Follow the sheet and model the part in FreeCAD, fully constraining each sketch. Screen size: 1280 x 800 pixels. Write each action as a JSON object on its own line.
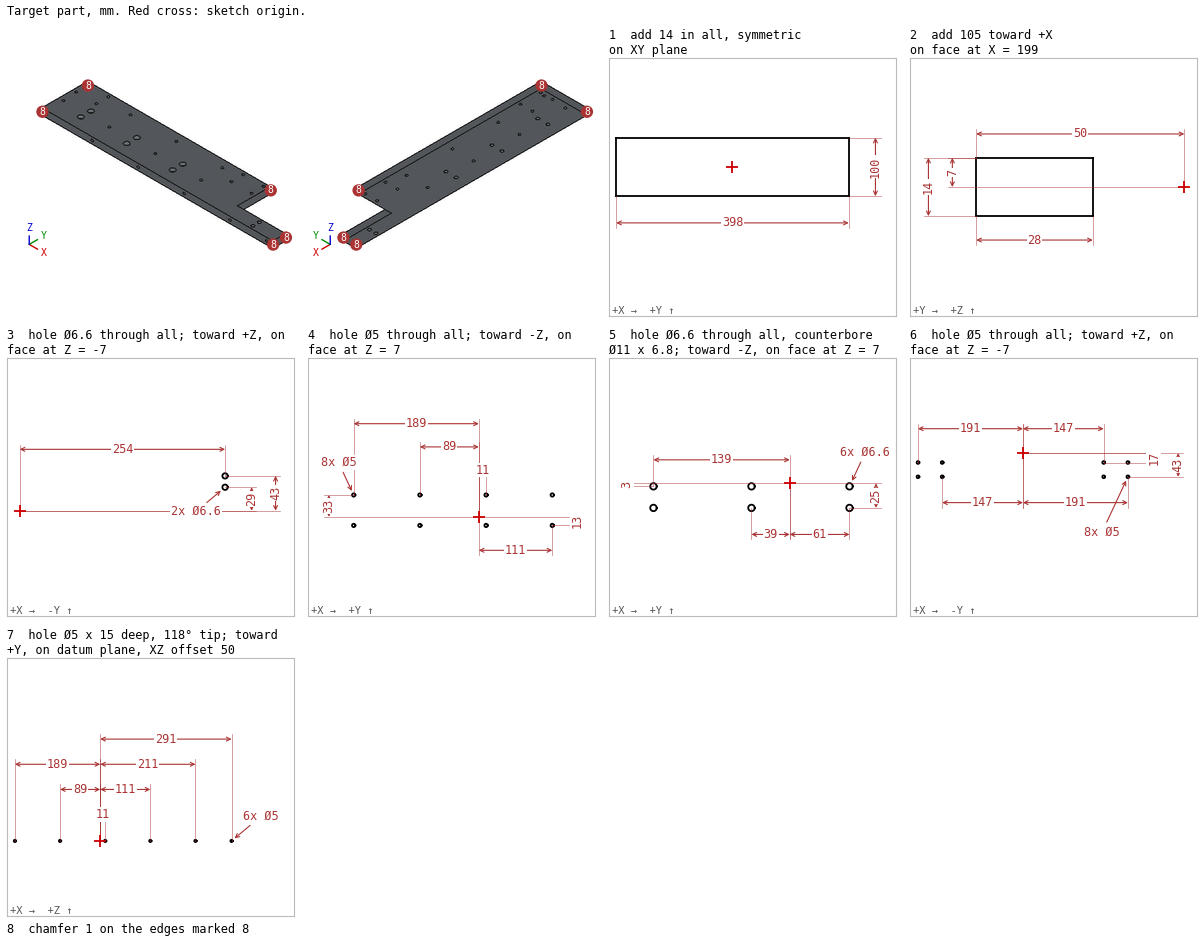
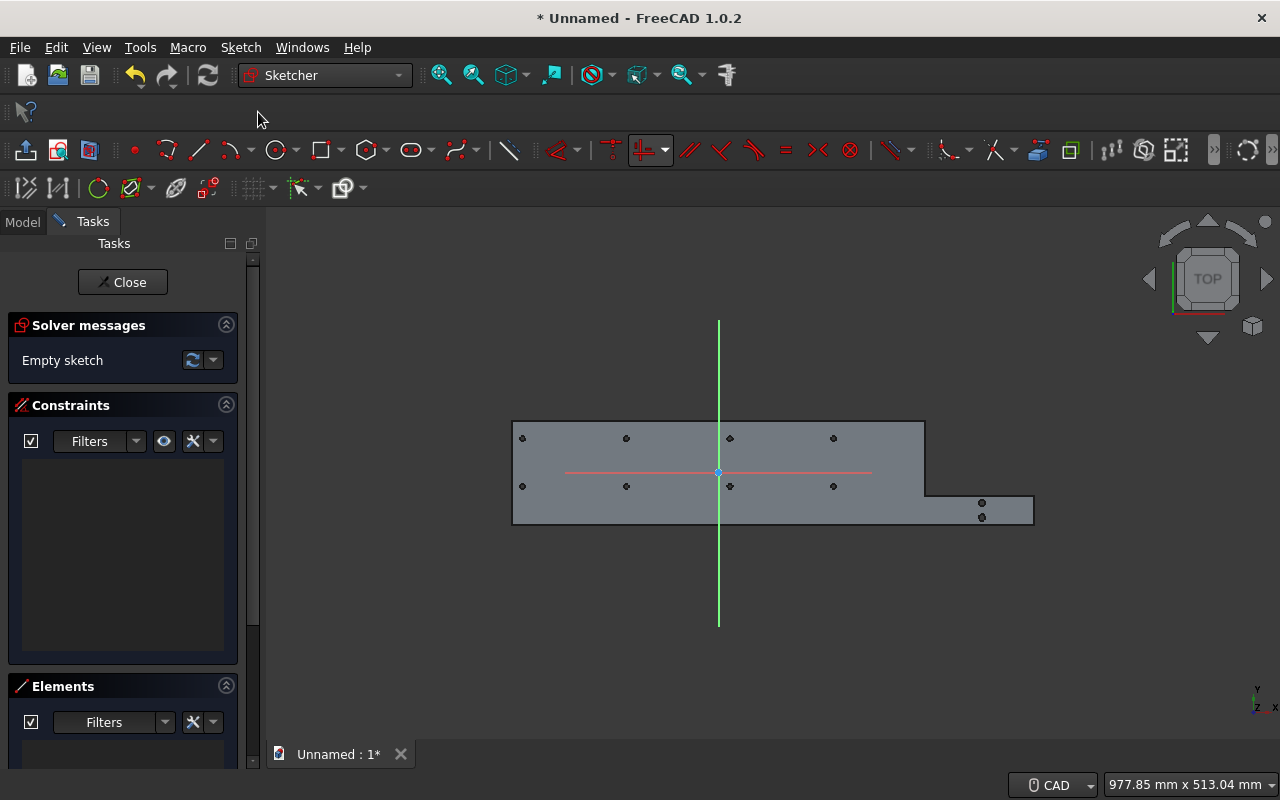
{"action": "scroll", "coordinate": [663, 496], "scroll_direction": "up", "scroll_amount": 5}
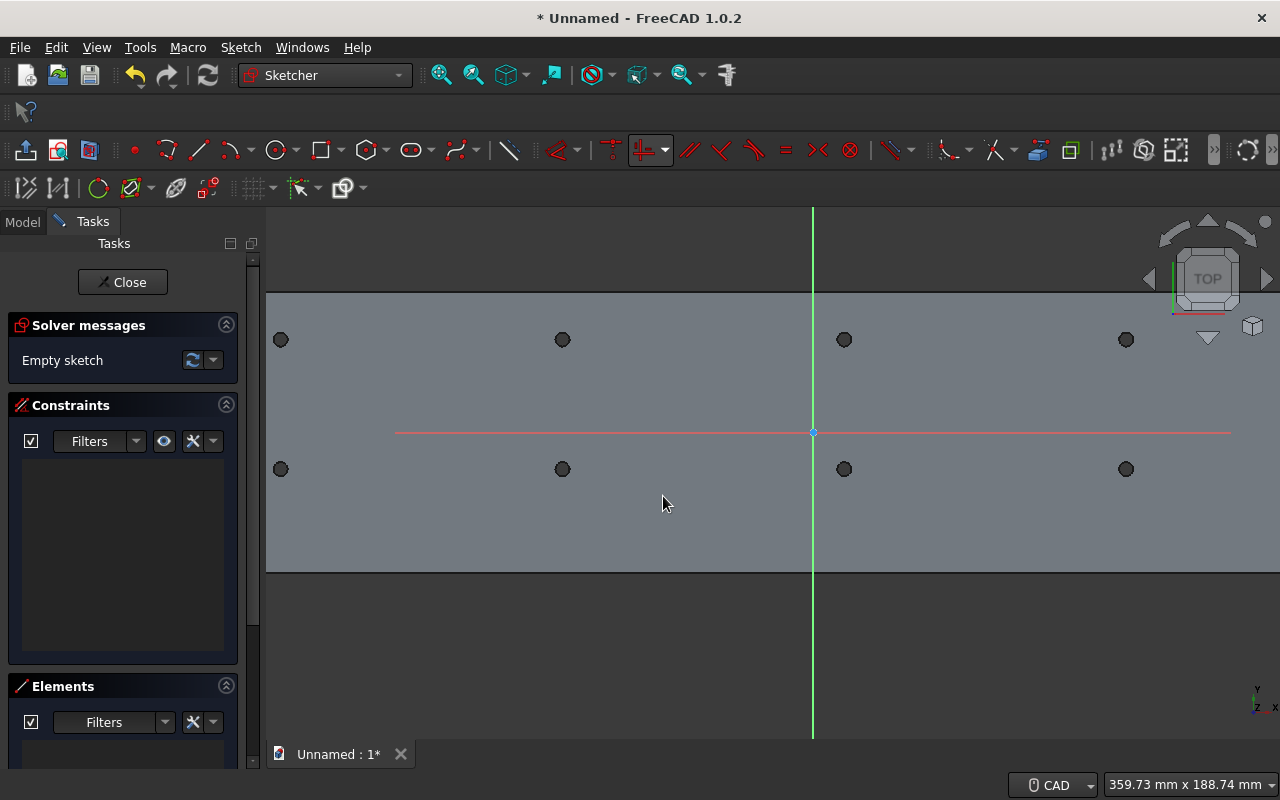
{"action": "left_click", "coordinate": [276, 150]}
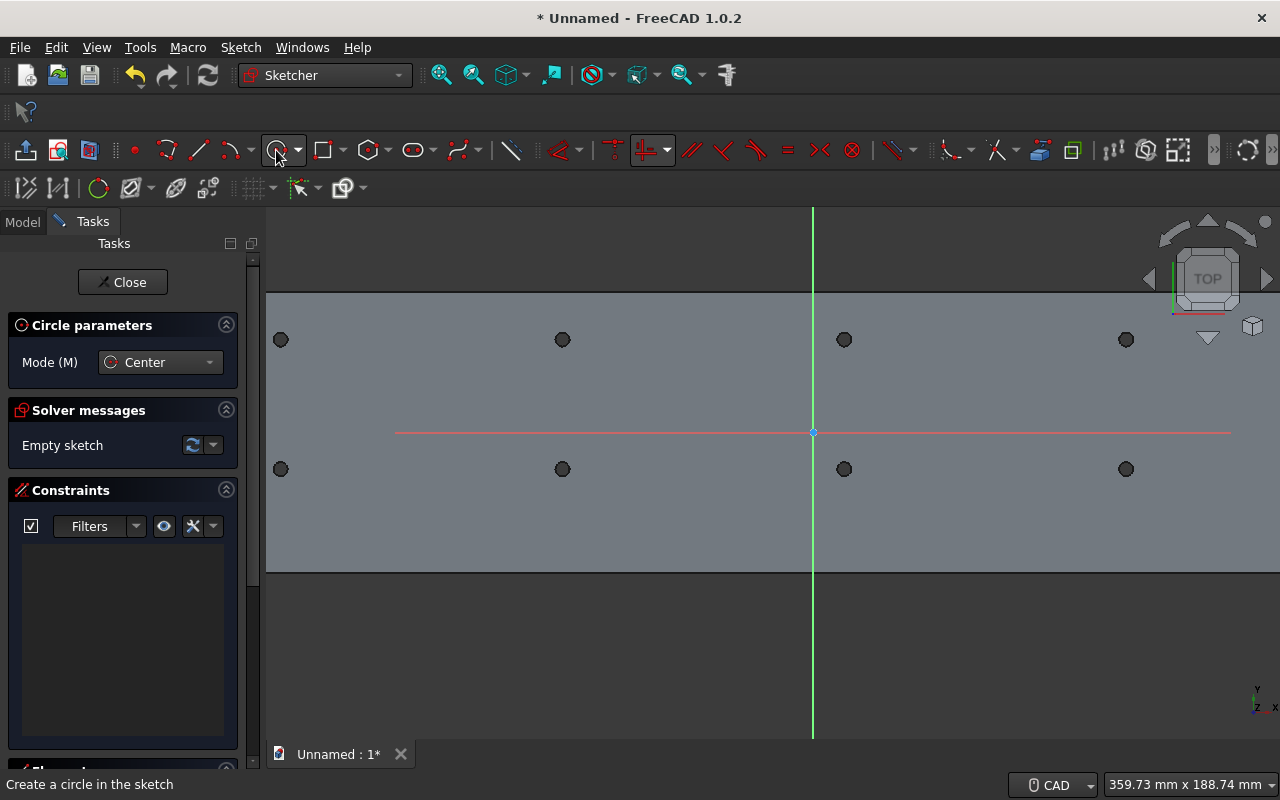
{"action": "scroll", "coordinate": [422, 441], "scroll_direction": "up", "scroll_amount": 5}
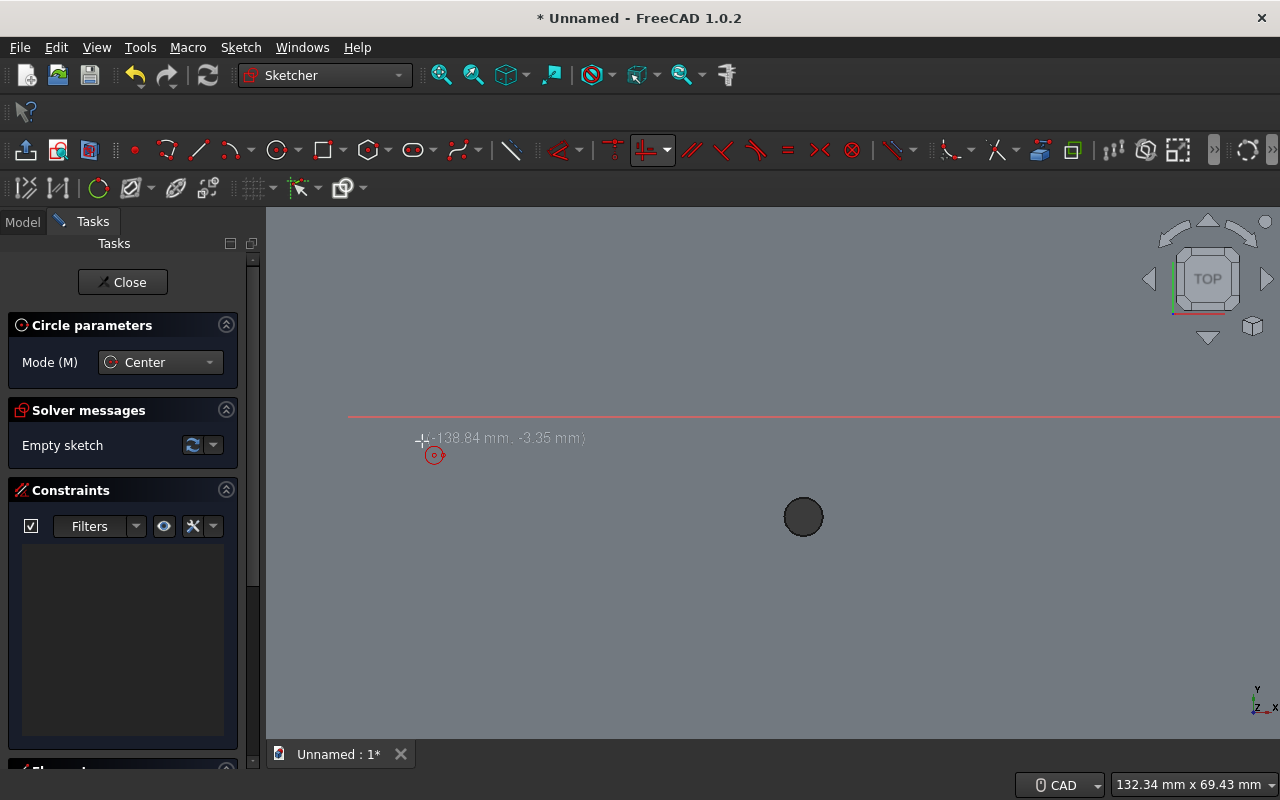
{"action": "left_click", "coordinate": [420, 440]}
{"action": "left_click", "coordinate": [438, 458]}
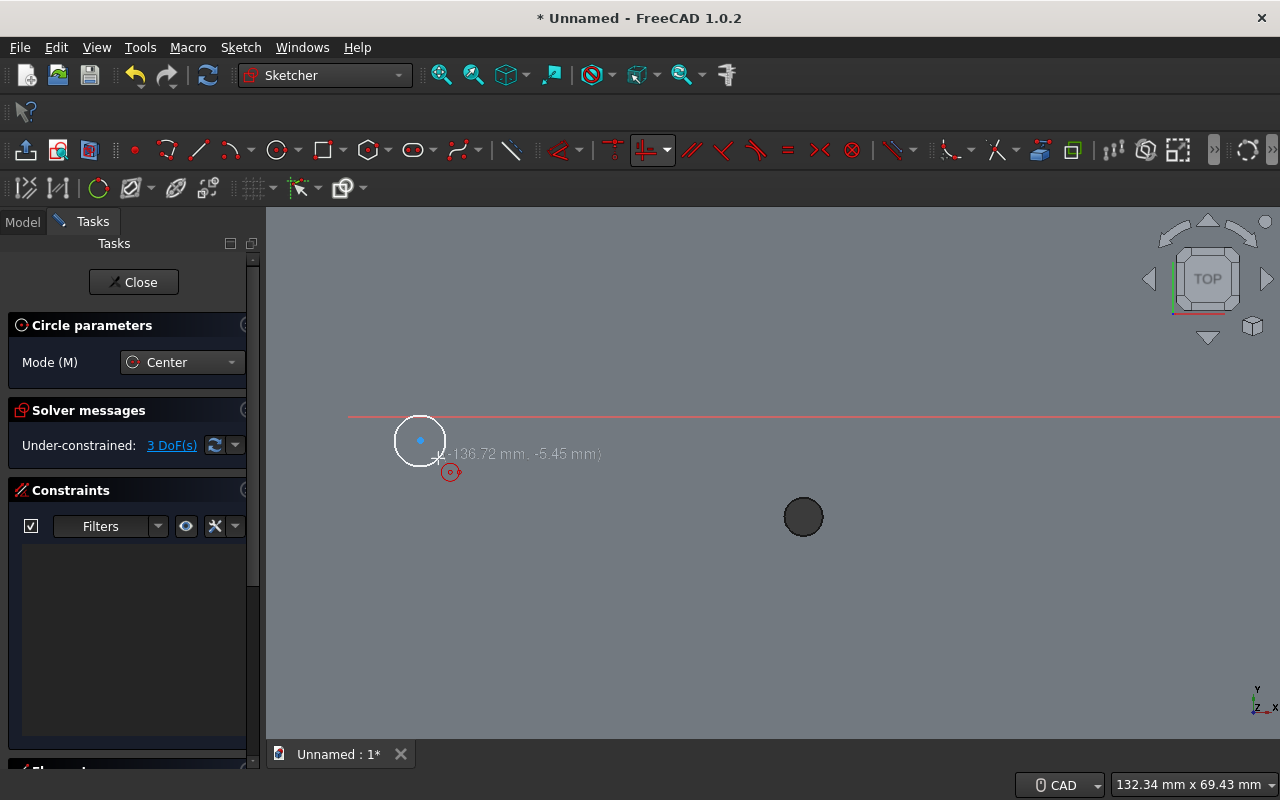
{"action": "scroll", "coordinate": [424, 443], "scroll_direction": "down", "scroll_amount": 5}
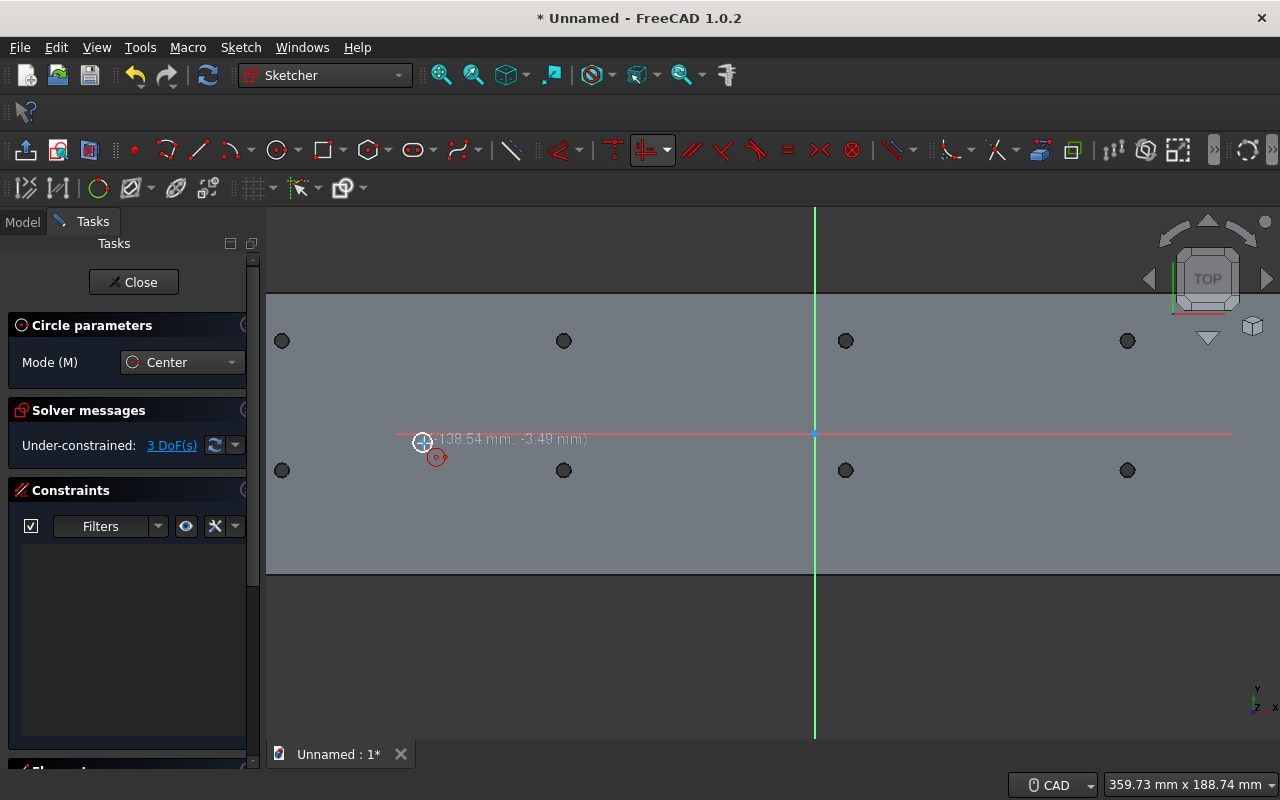
{"action": "scroll", "coordinate": [987, 504], "scroll_direction": "up", "scroll_amount": 5}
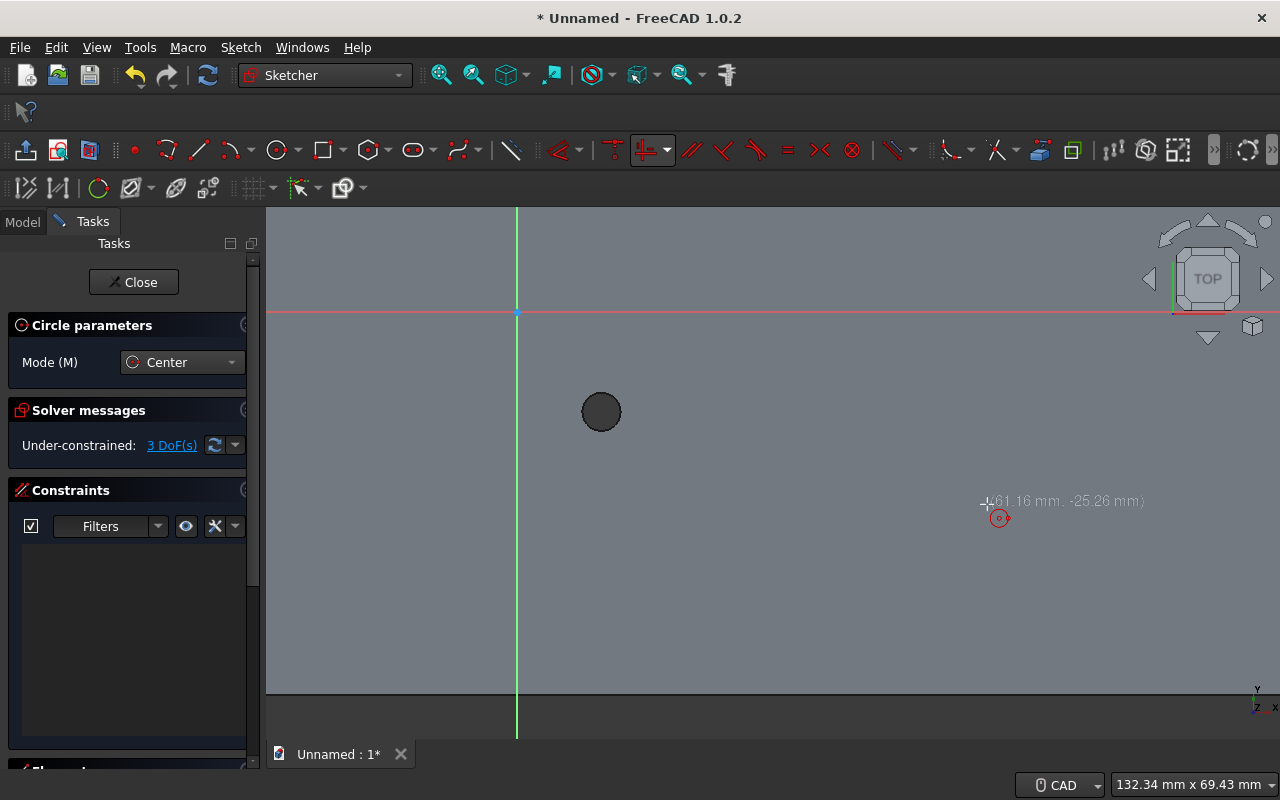
{"action": "left_click", "coordinate": [985, 504]}
{"action": "left_click", "coordinate": [1002, 486]}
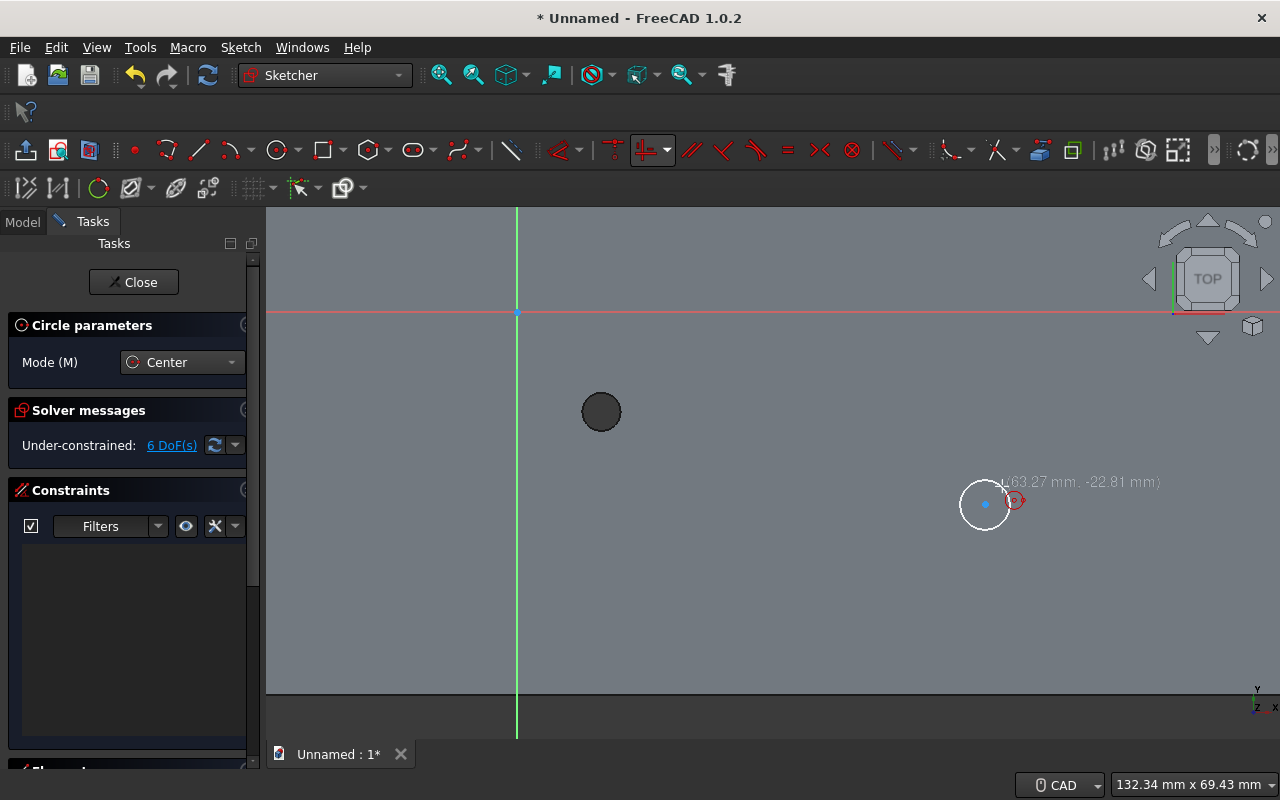
{"action": "left_click", "coordinate": [985, 335]}
{"action": "left_click", "coordinate": [1002, 353]}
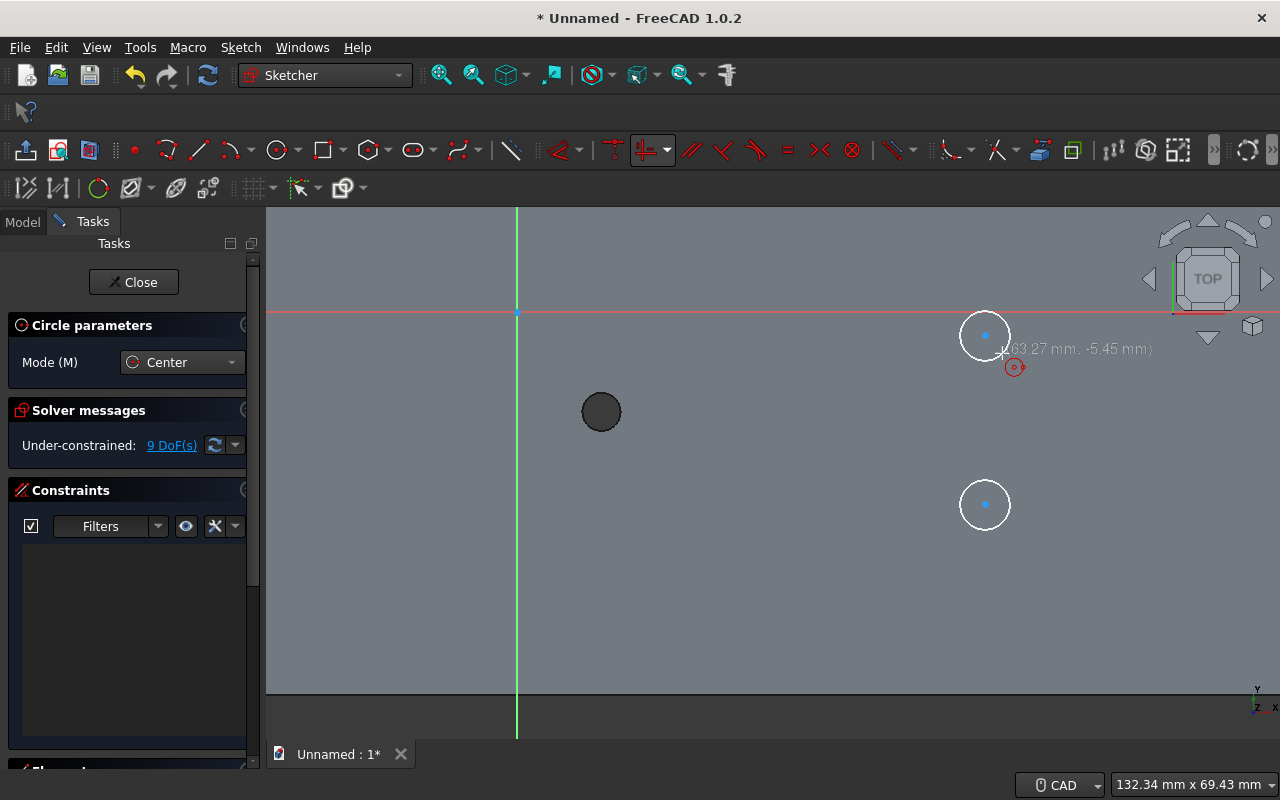
{"action": "scroll", "coordinate": [987, 504], "scroll_direction": "down", "scroll_amount": 5}